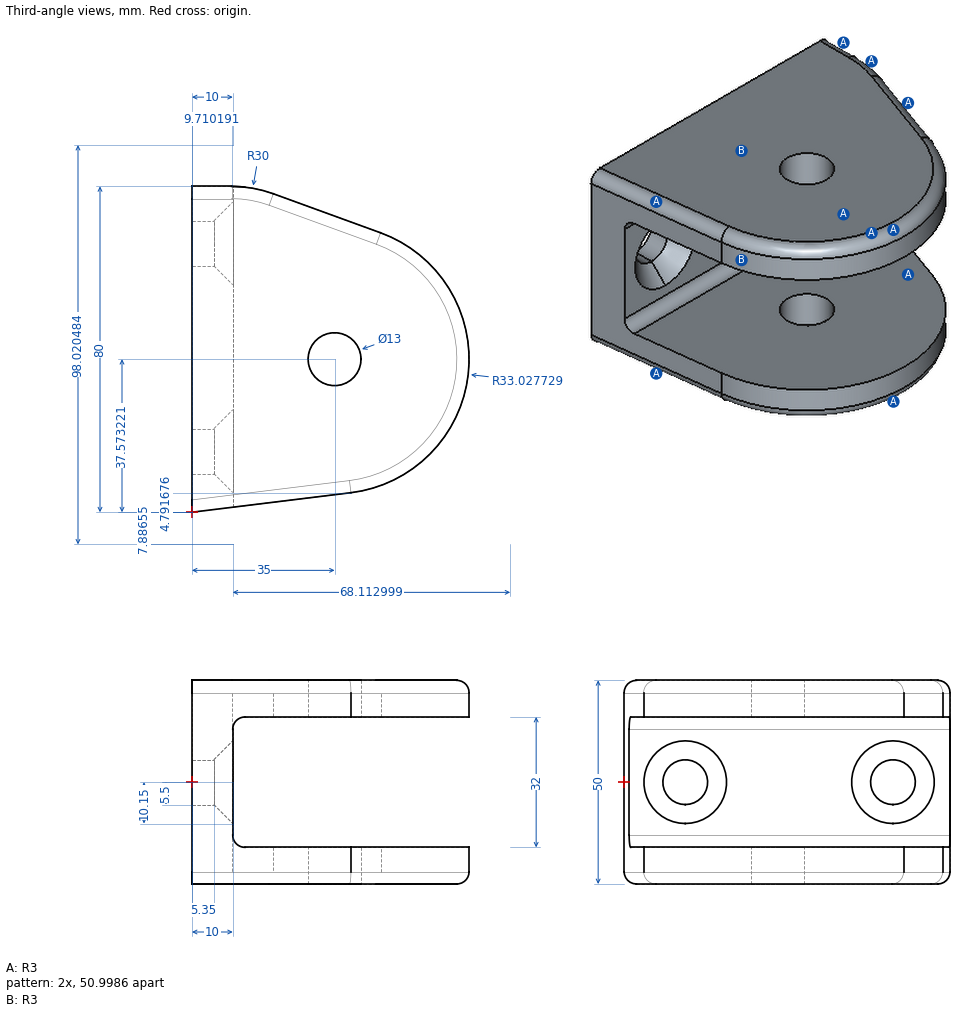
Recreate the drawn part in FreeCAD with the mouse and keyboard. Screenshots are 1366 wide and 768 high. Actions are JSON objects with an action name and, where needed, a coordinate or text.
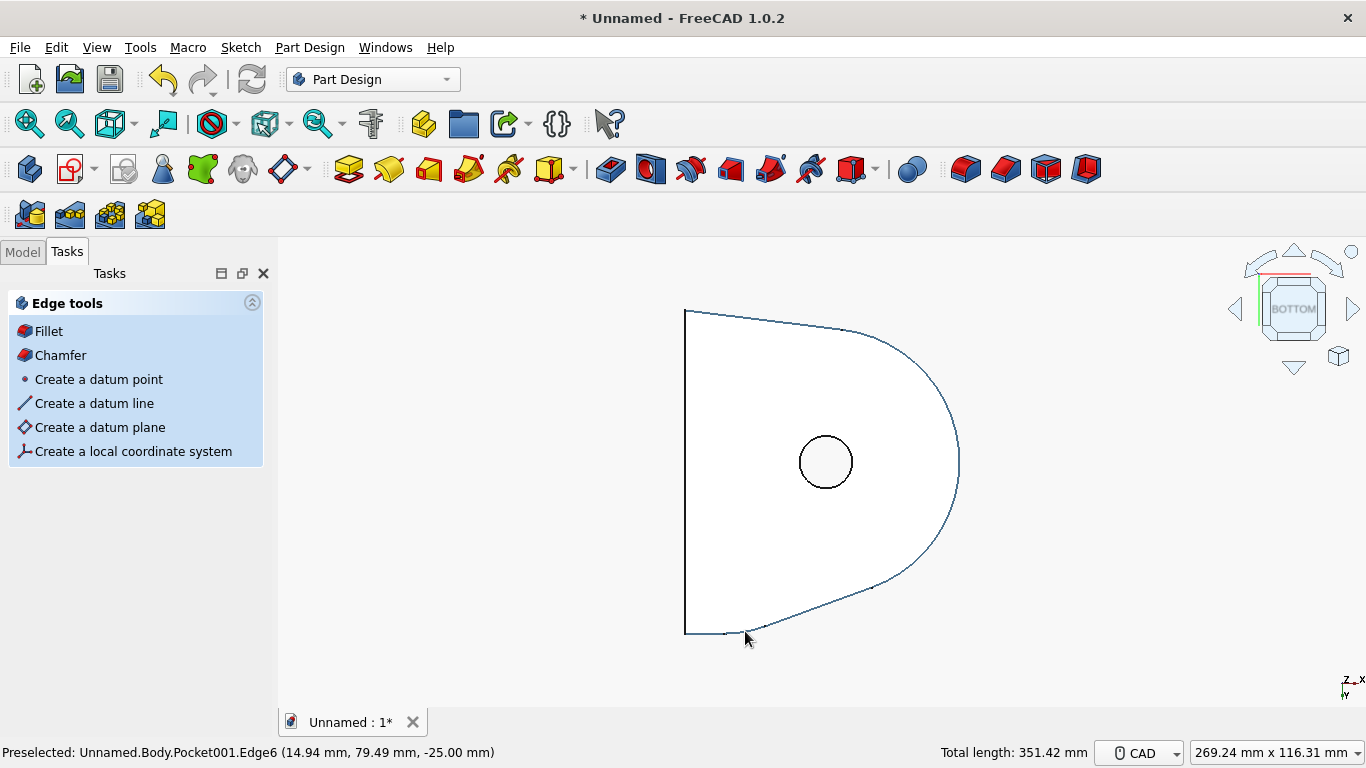
{"action": "left_click", "coordinate": [966, 170]}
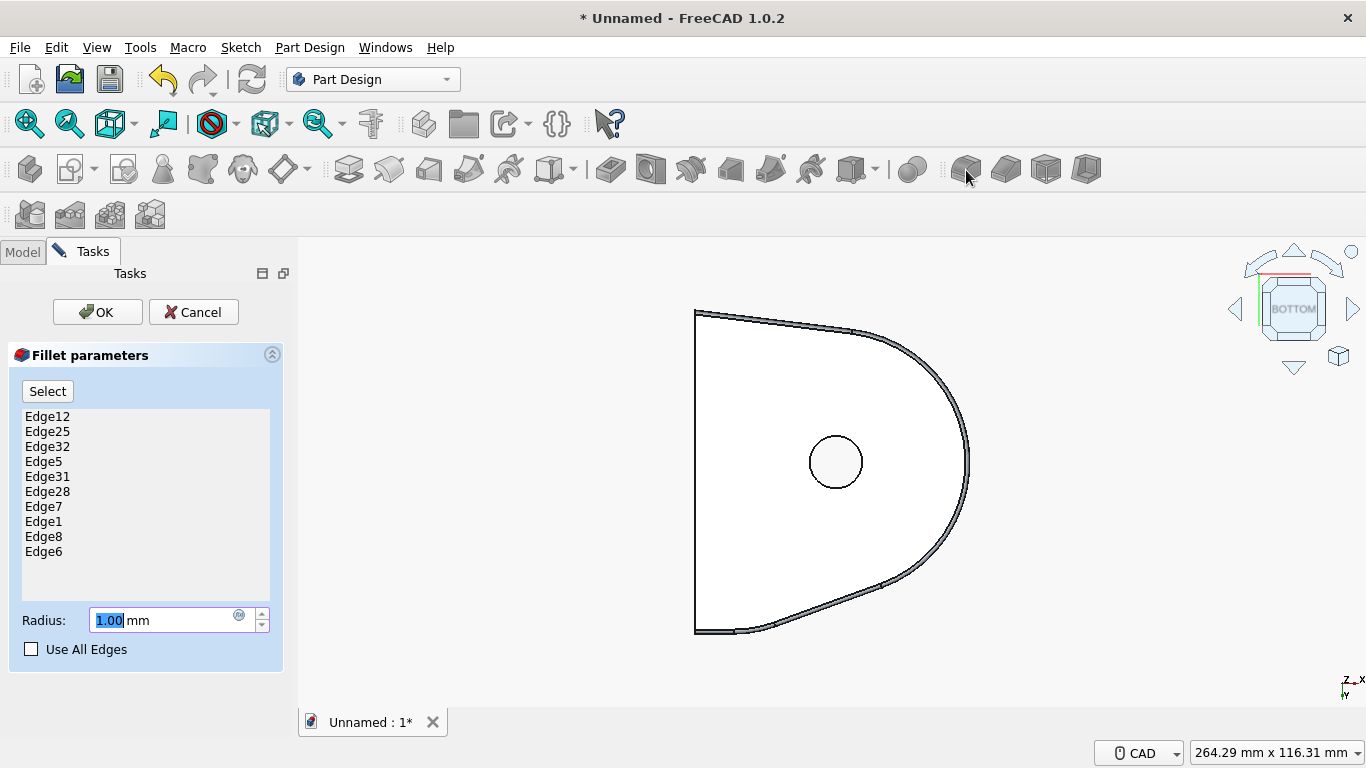
{"action": "type", "text": "3"}
{"action": "key", "text": "Tab"}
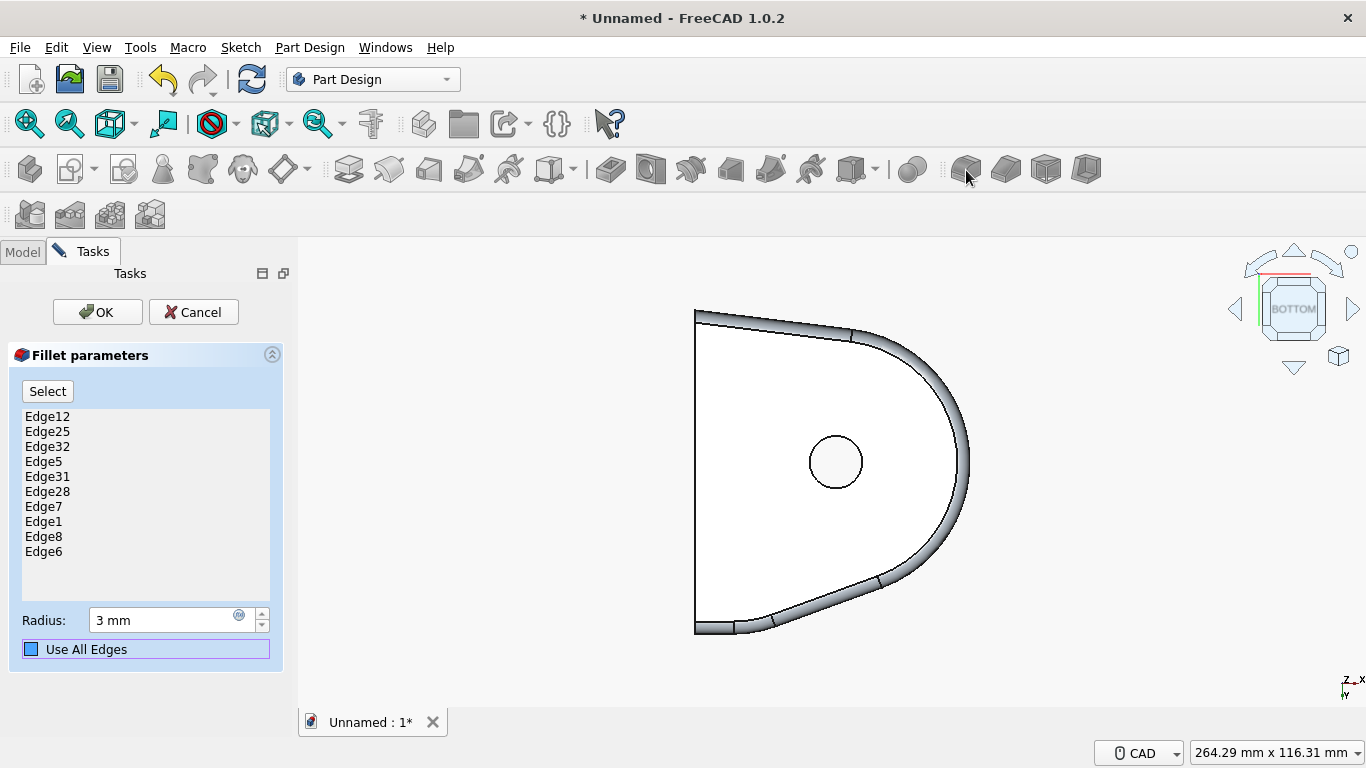
{"action": "left_click", "coordinate": [98, 312]}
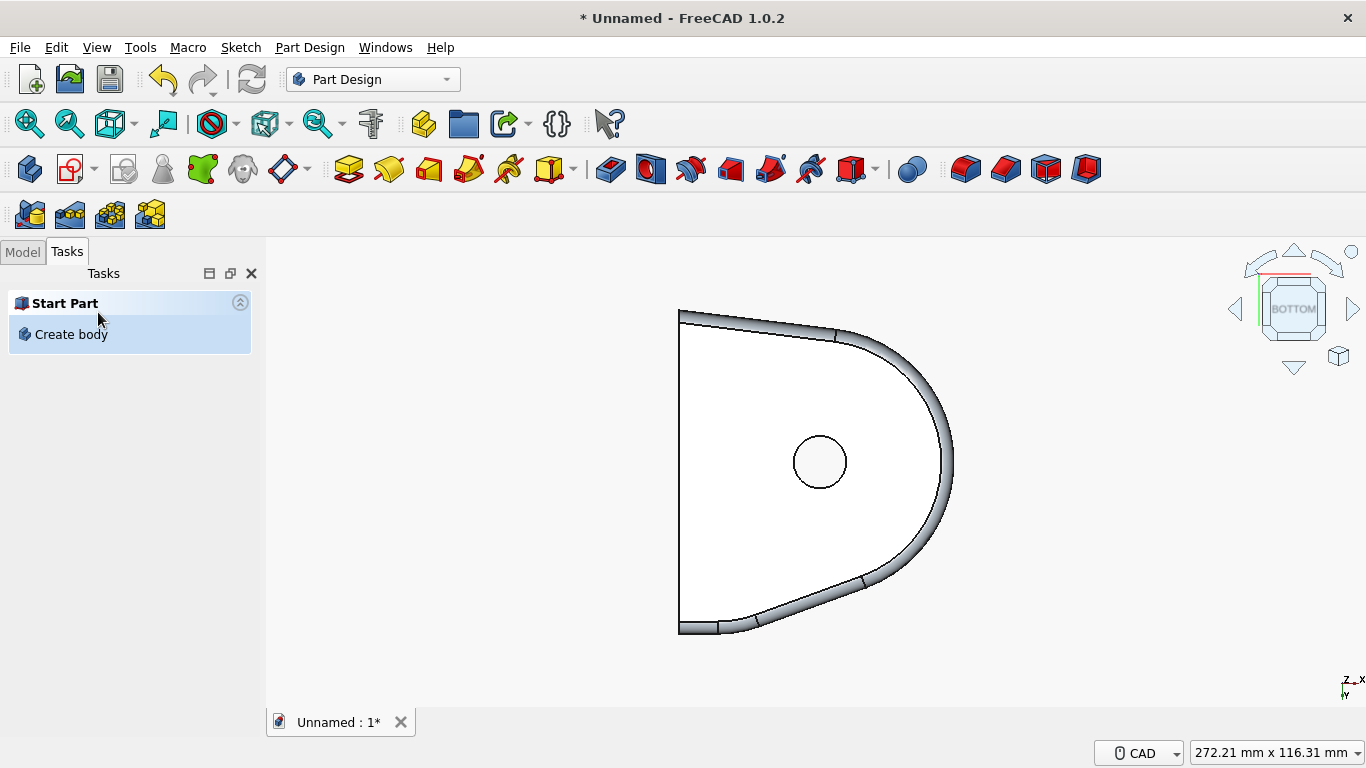
{"action": "left_click", "coordinate": [23, 251]}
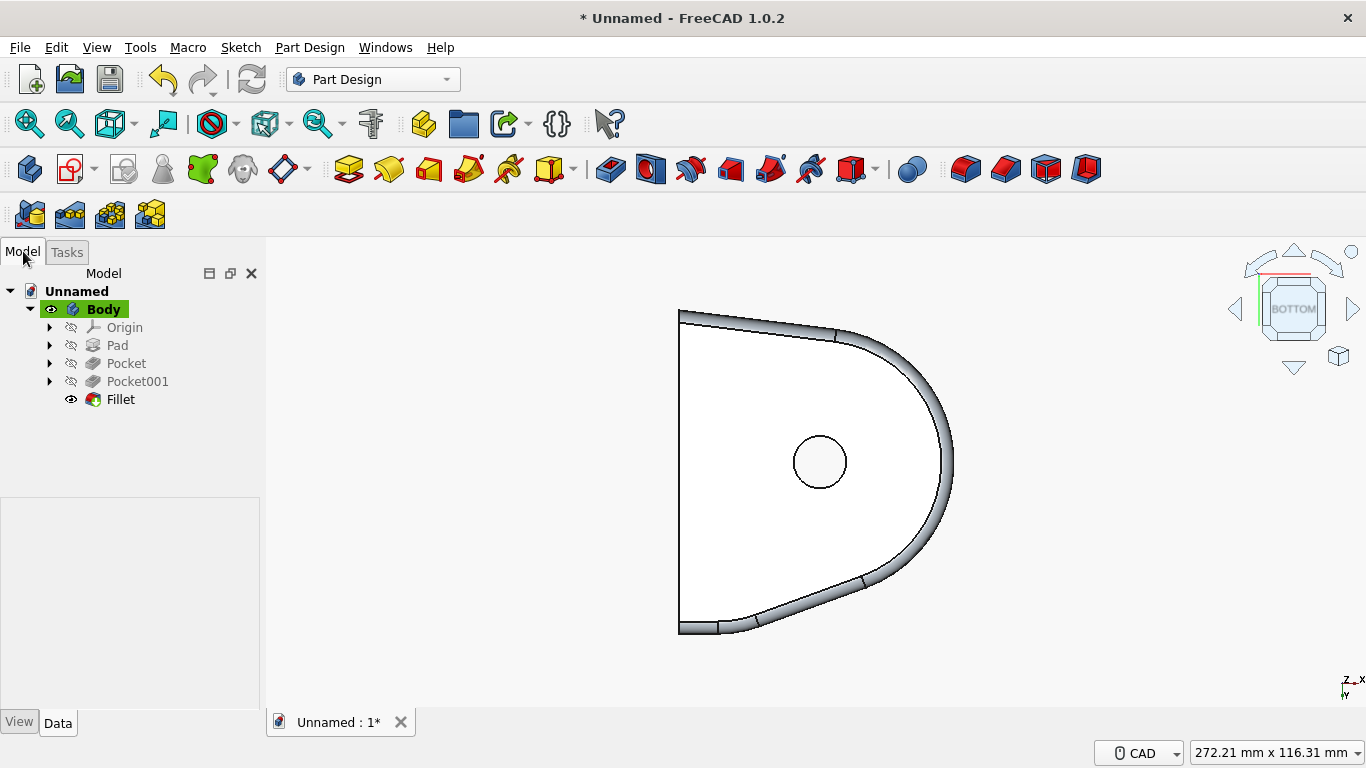
{"action": "left_click", "coordinate": [50, 327]}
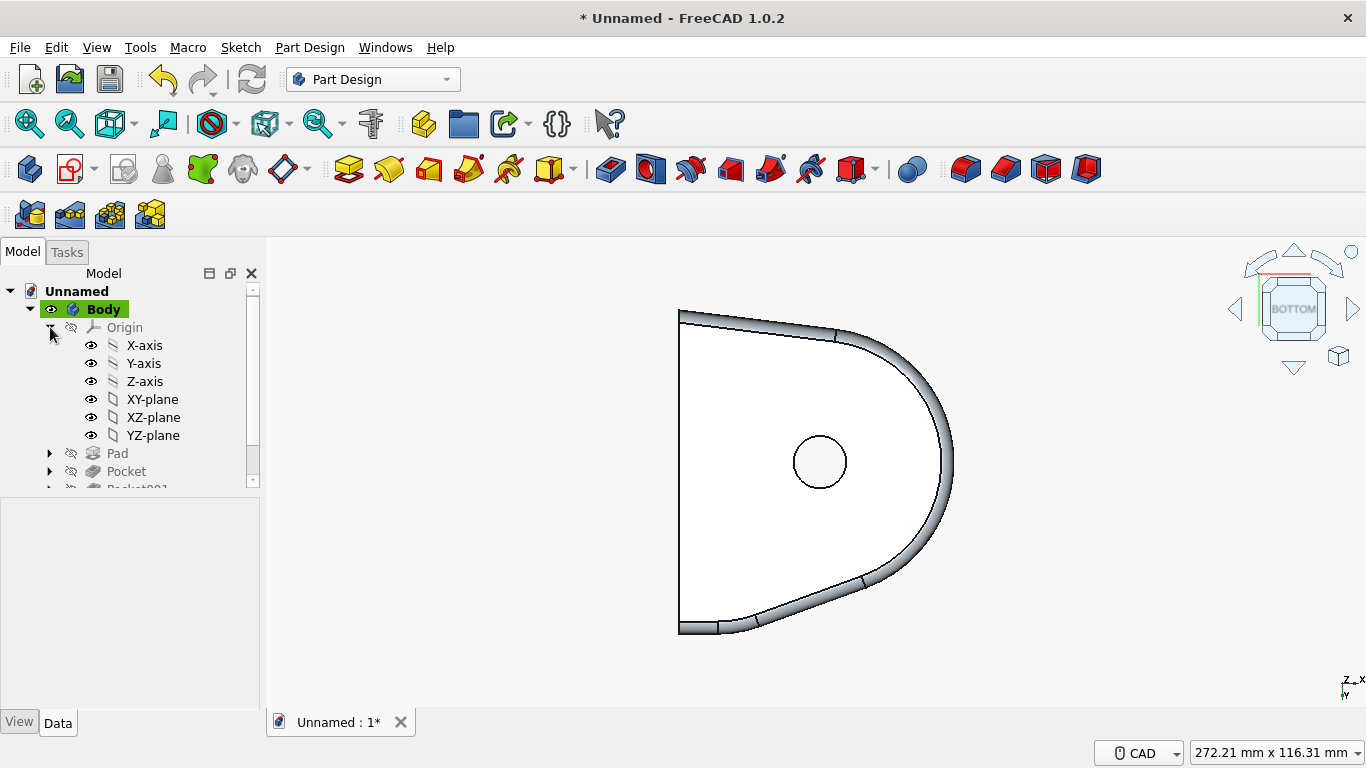
{"action": "left_click", "coordinate": [136, 417]}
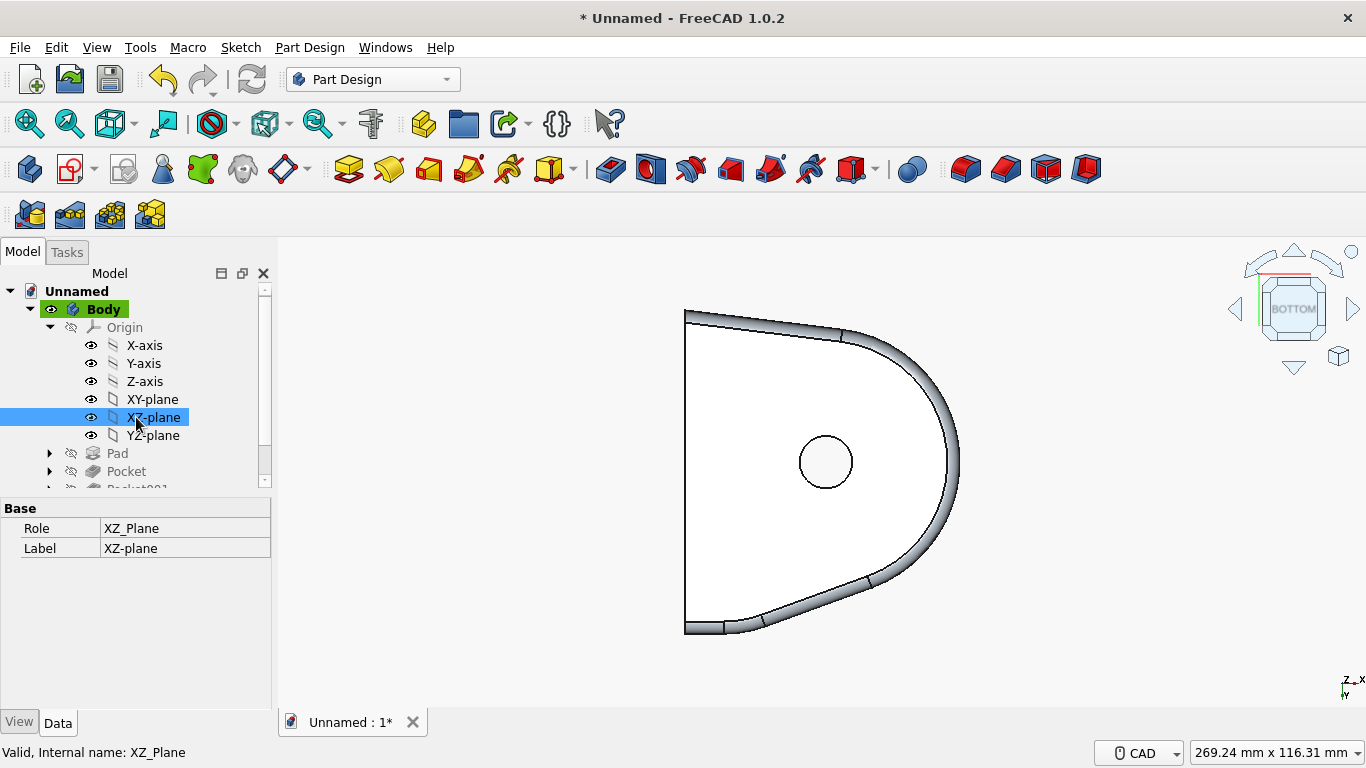
{"action": "left_click", "coordinate": [284, 170]}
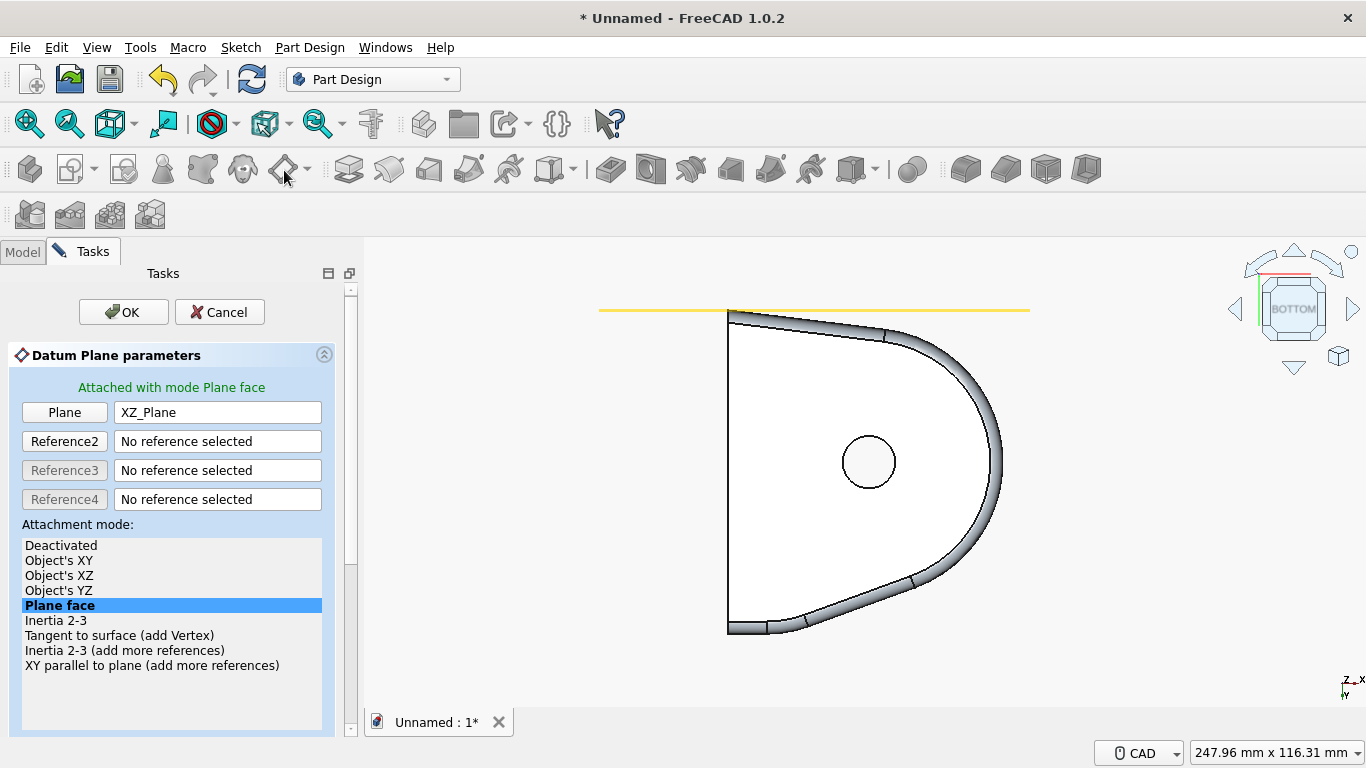
{"action": "scroll", "coordinate": [351, 510], "scroll_direction": "down", "scroll_amount": 3}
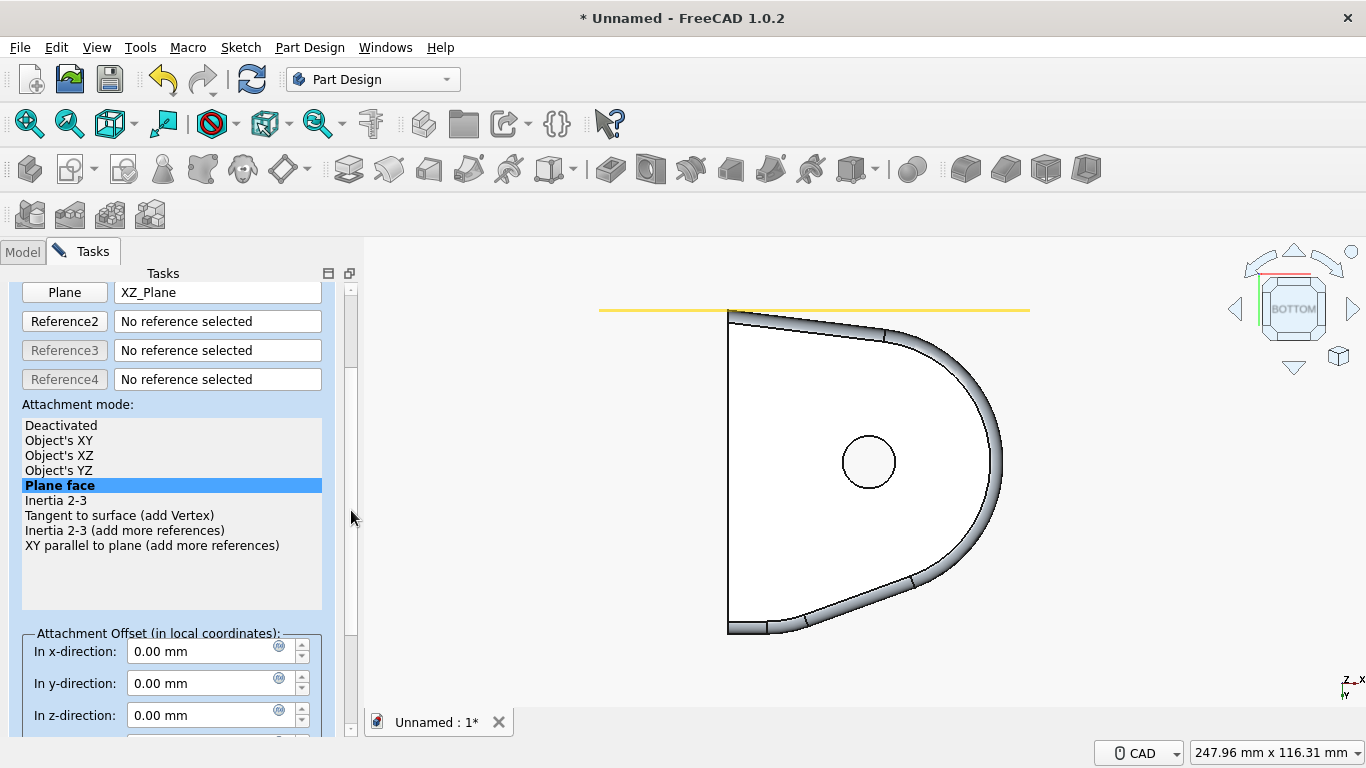
{"action": "triple_click", "coordinate": [210, 655]}